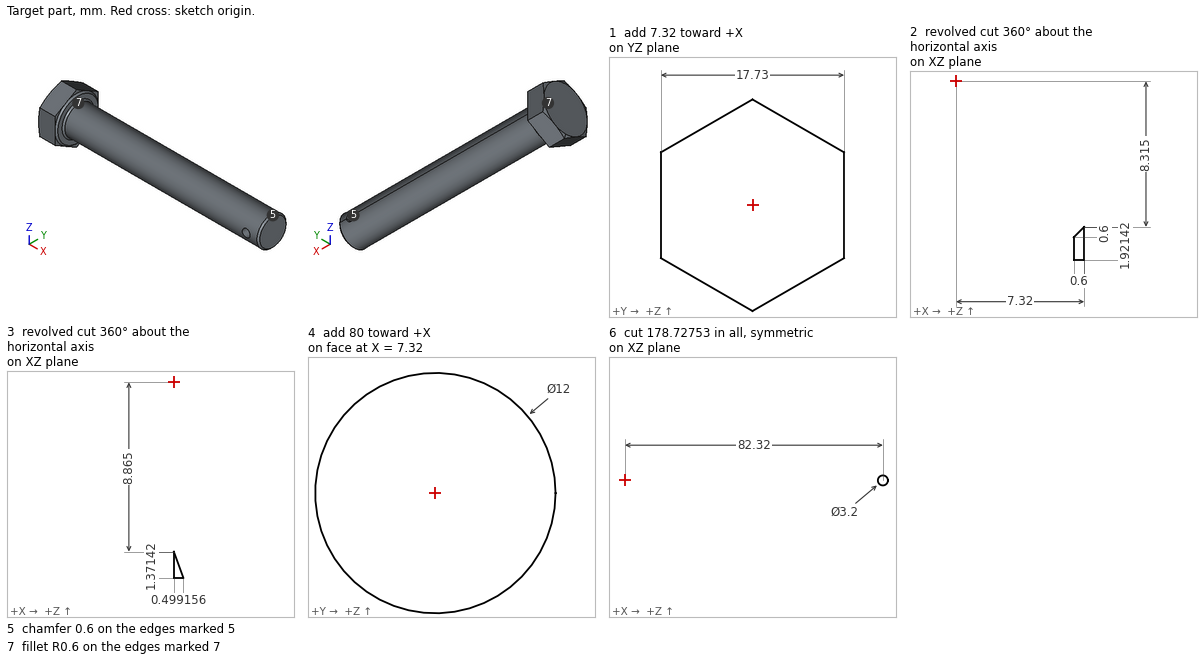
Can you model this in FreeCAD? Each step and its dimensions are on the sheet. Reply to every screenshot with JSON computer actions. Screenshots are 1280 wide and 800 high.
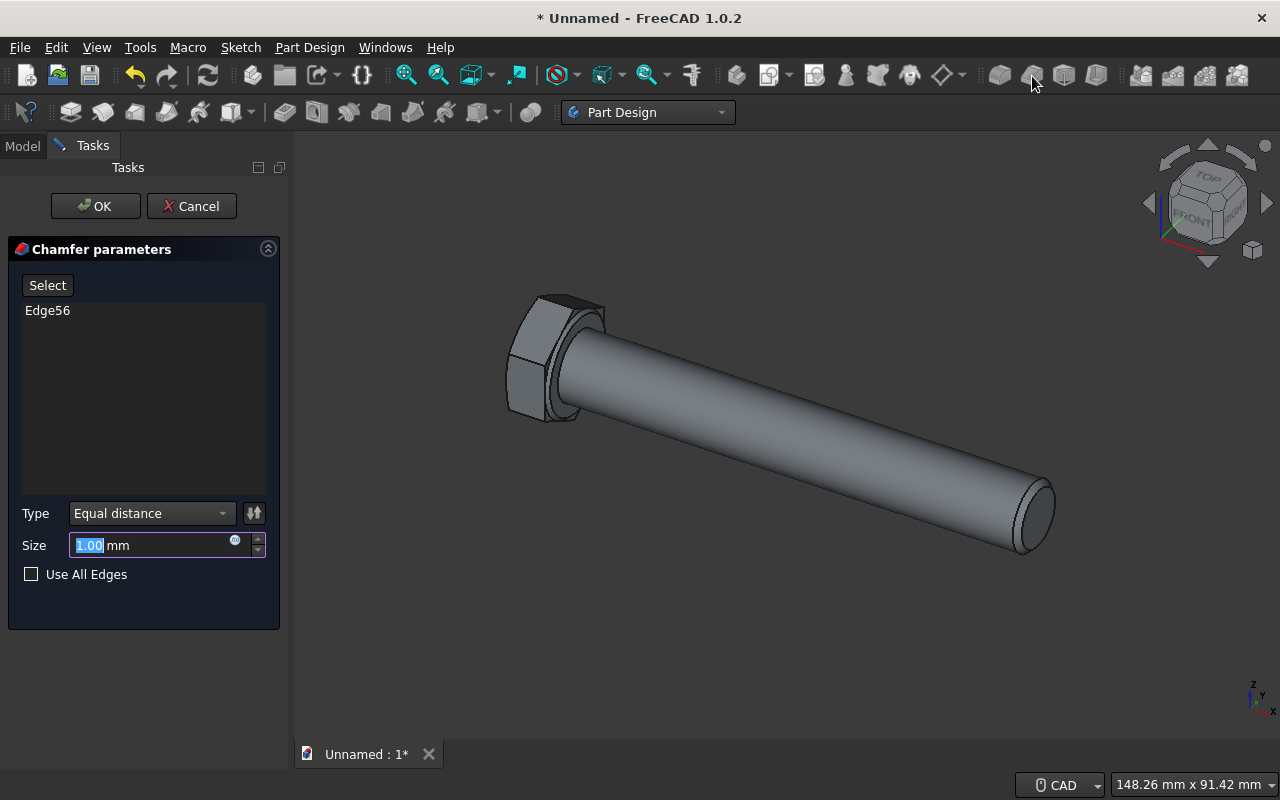
{"action": "type", "text": "0.6"}
{"action": "key", "text": "Tab"}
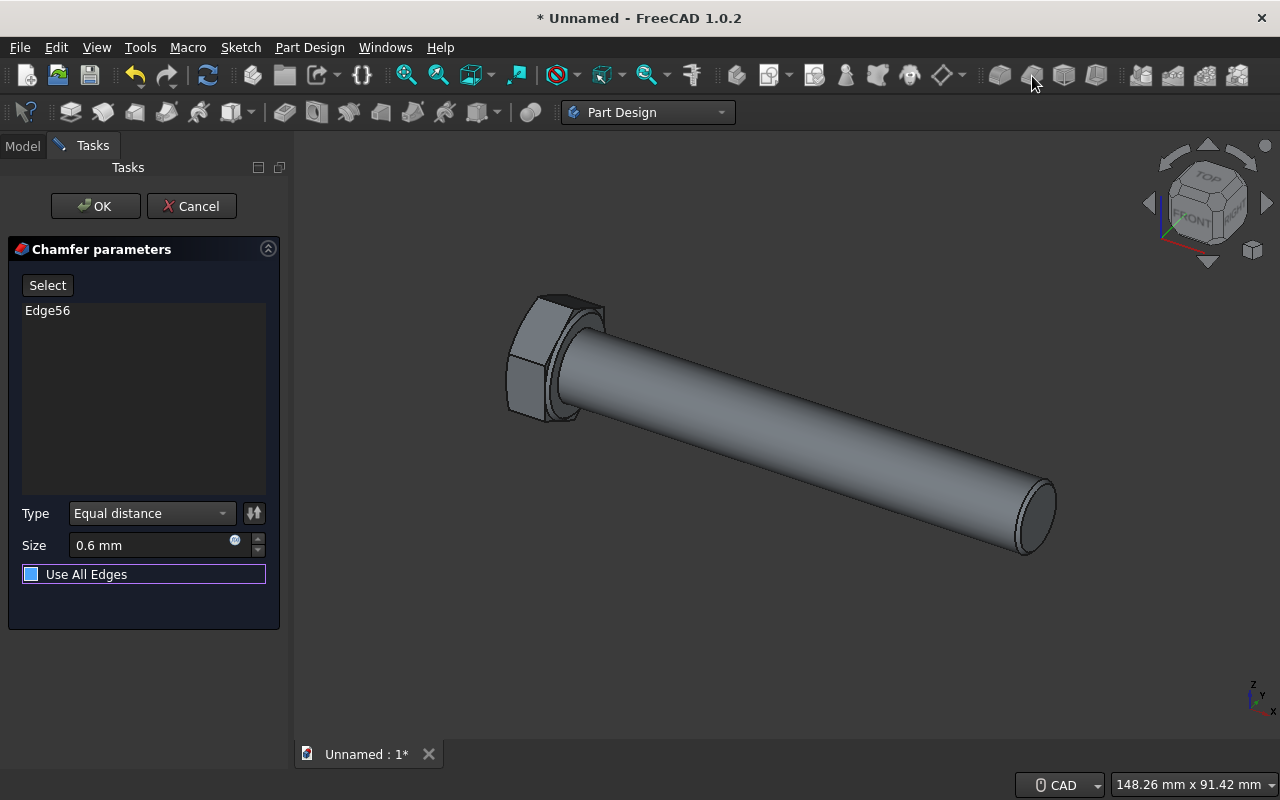
{"action": "left_click", "coordinate": [96, 206]}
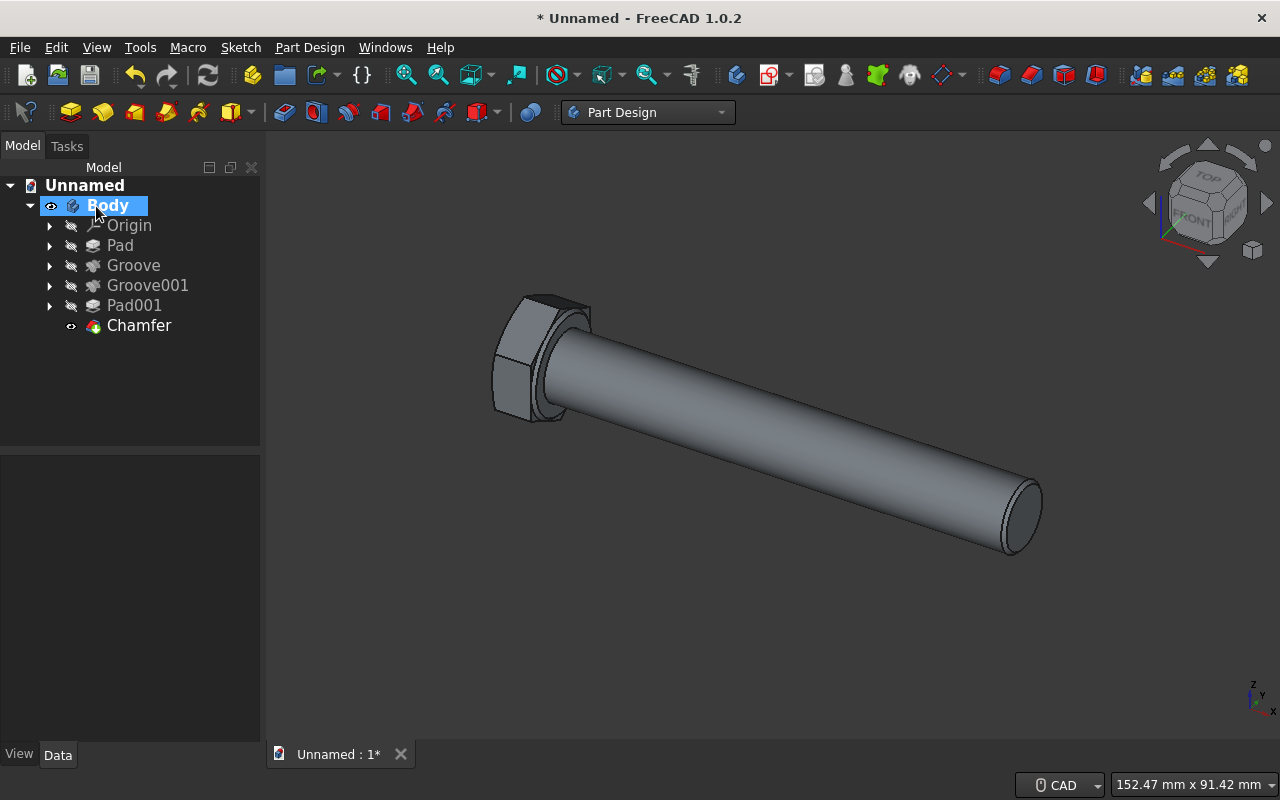
{"action": "left_click", "coordinate": [770, 76]}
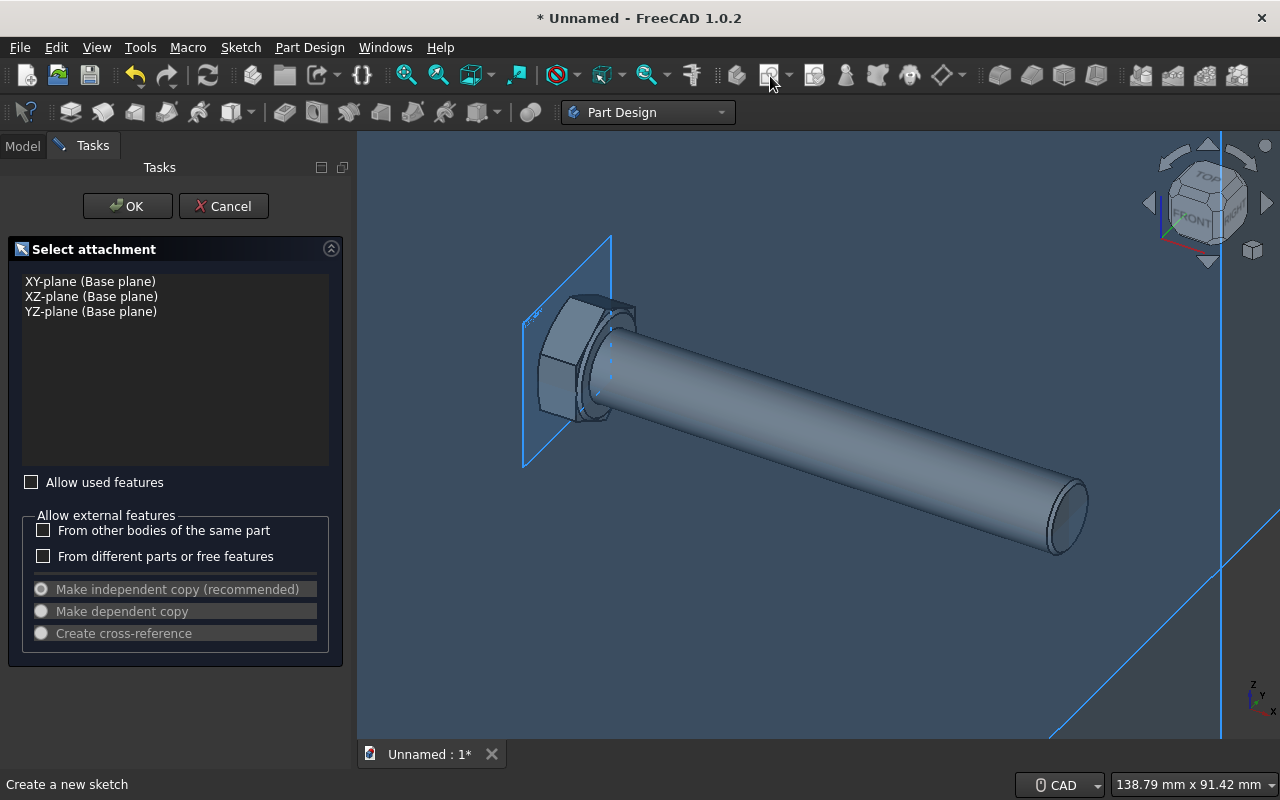
{"action": "left_click", "coordinate": [82, 296]}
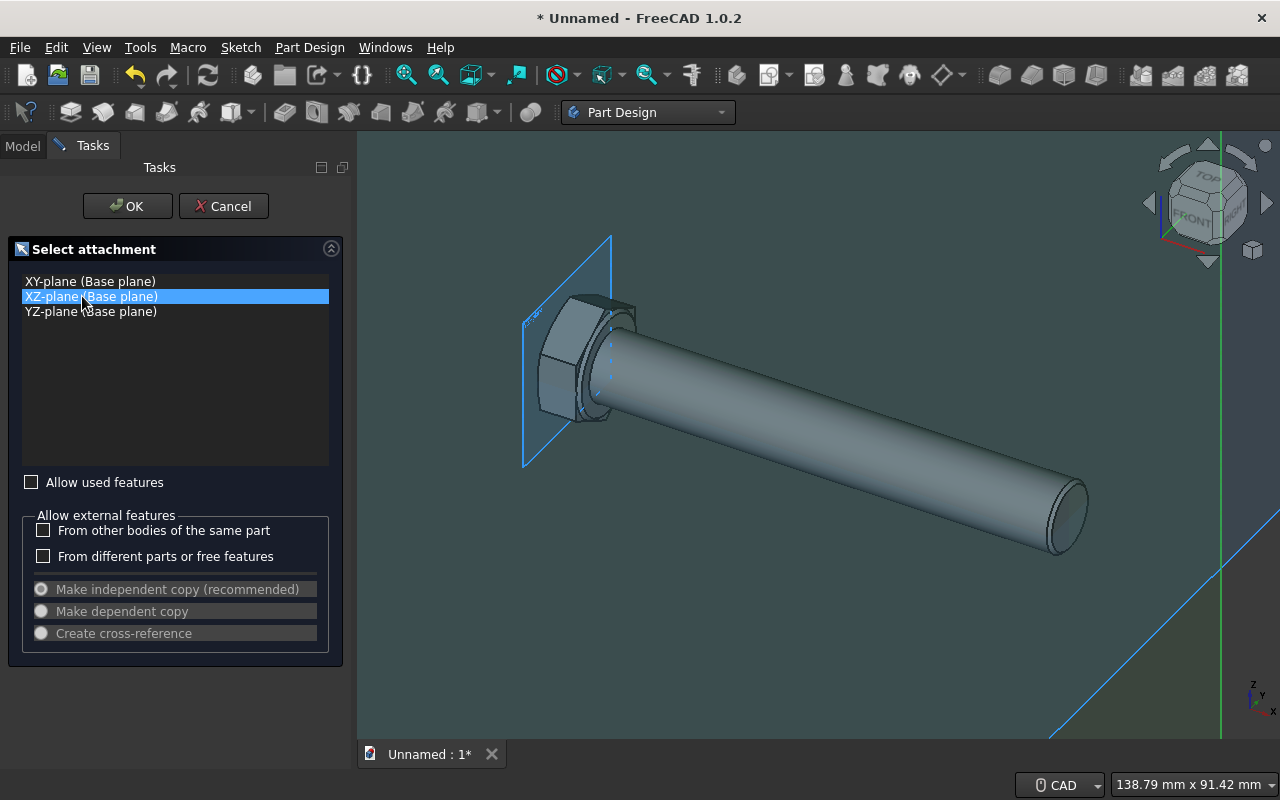
{"action": "left_click", "coordinate": [128, 206]}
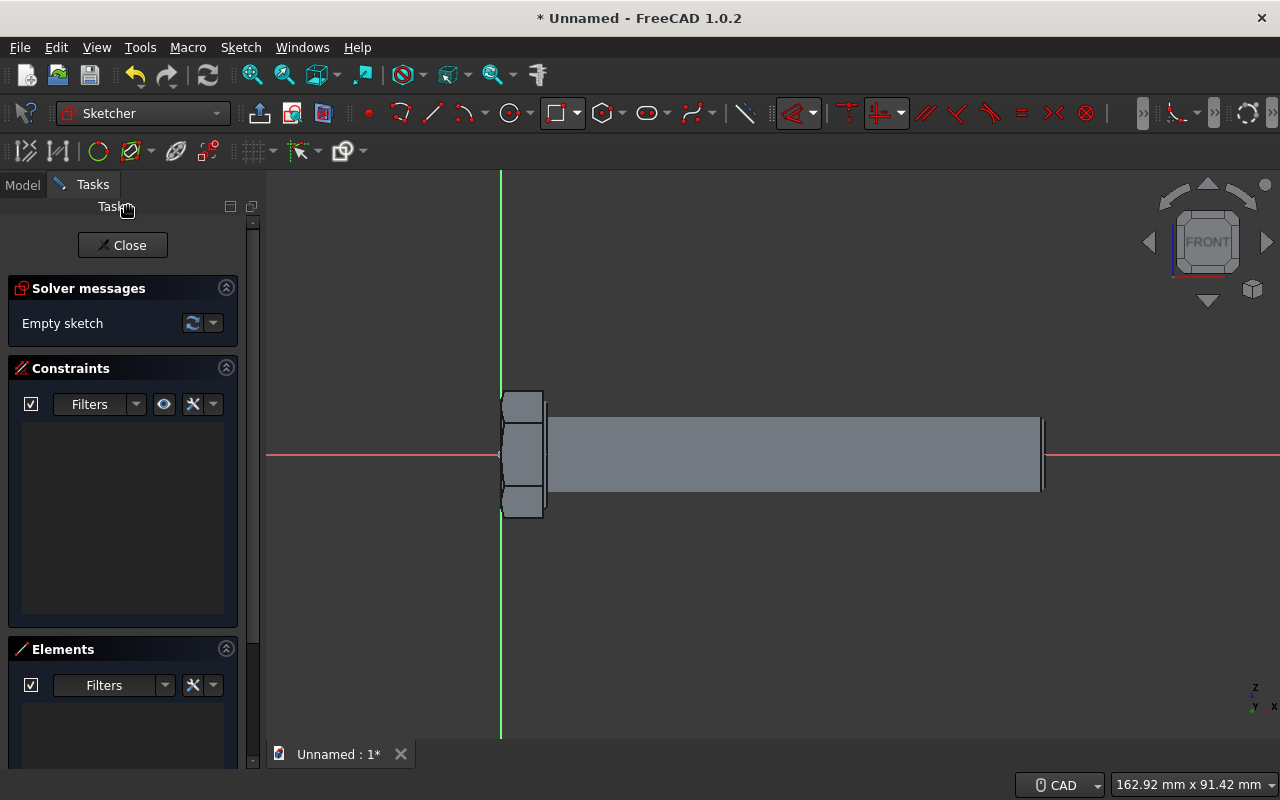
{"action": "left_click", "coordinate": [324, 114]}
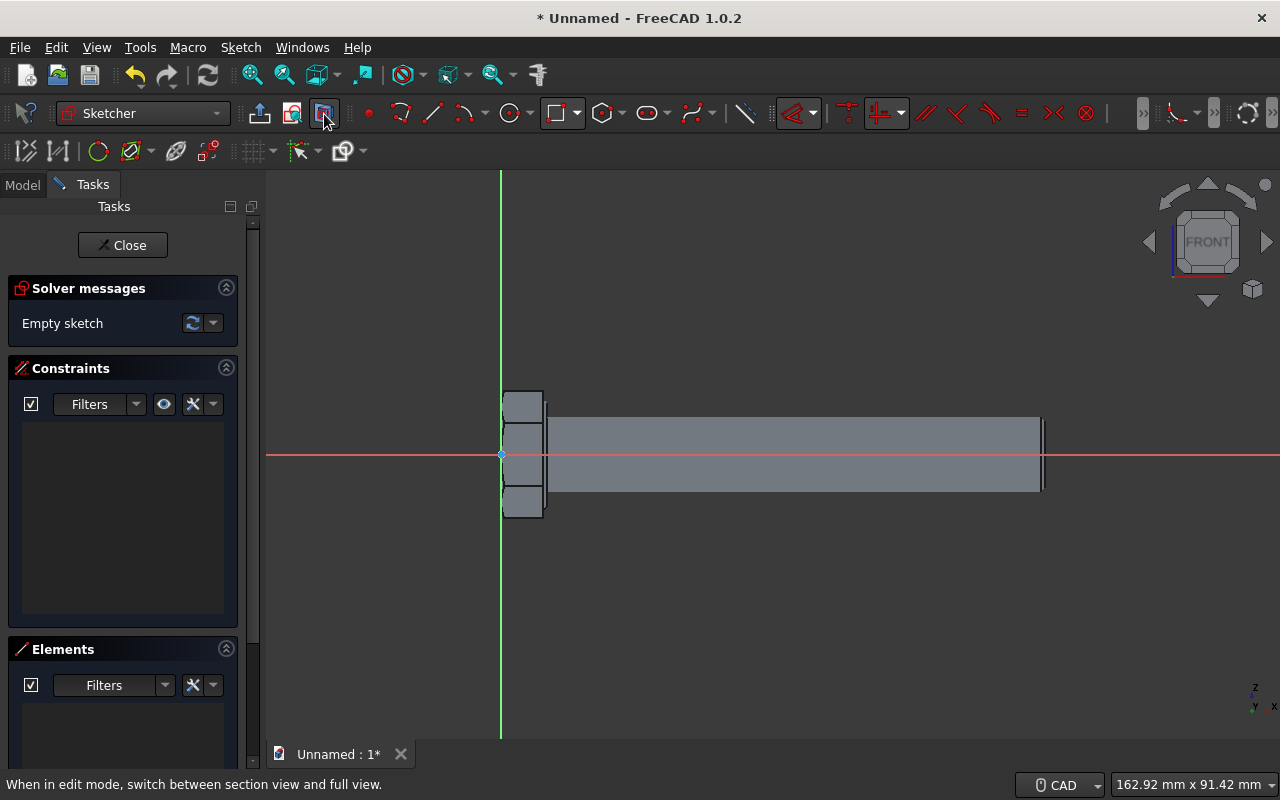
{"action": "scroll", "coordinate": [1030, 455], "scroll_direction": "up", "scroll_amount": 15}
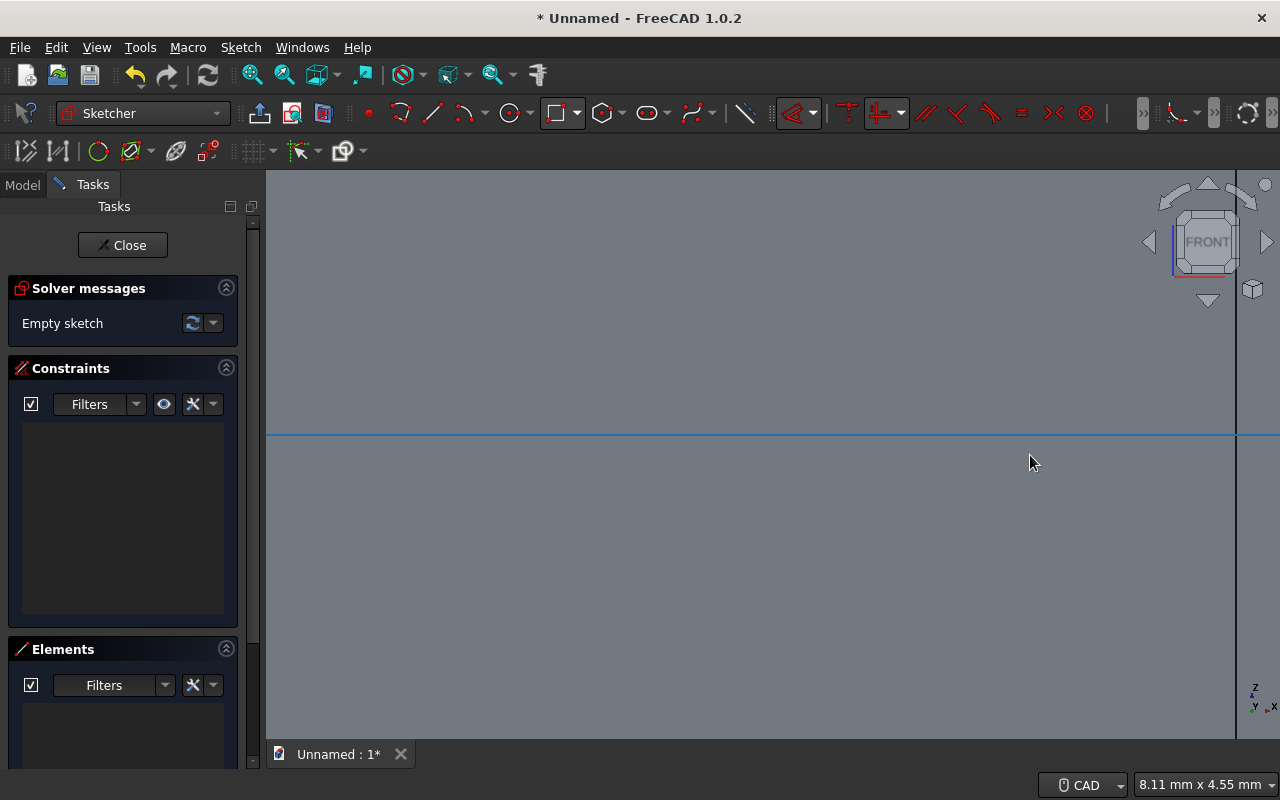
{"action": "left_click", "coordinate": [510, 114]}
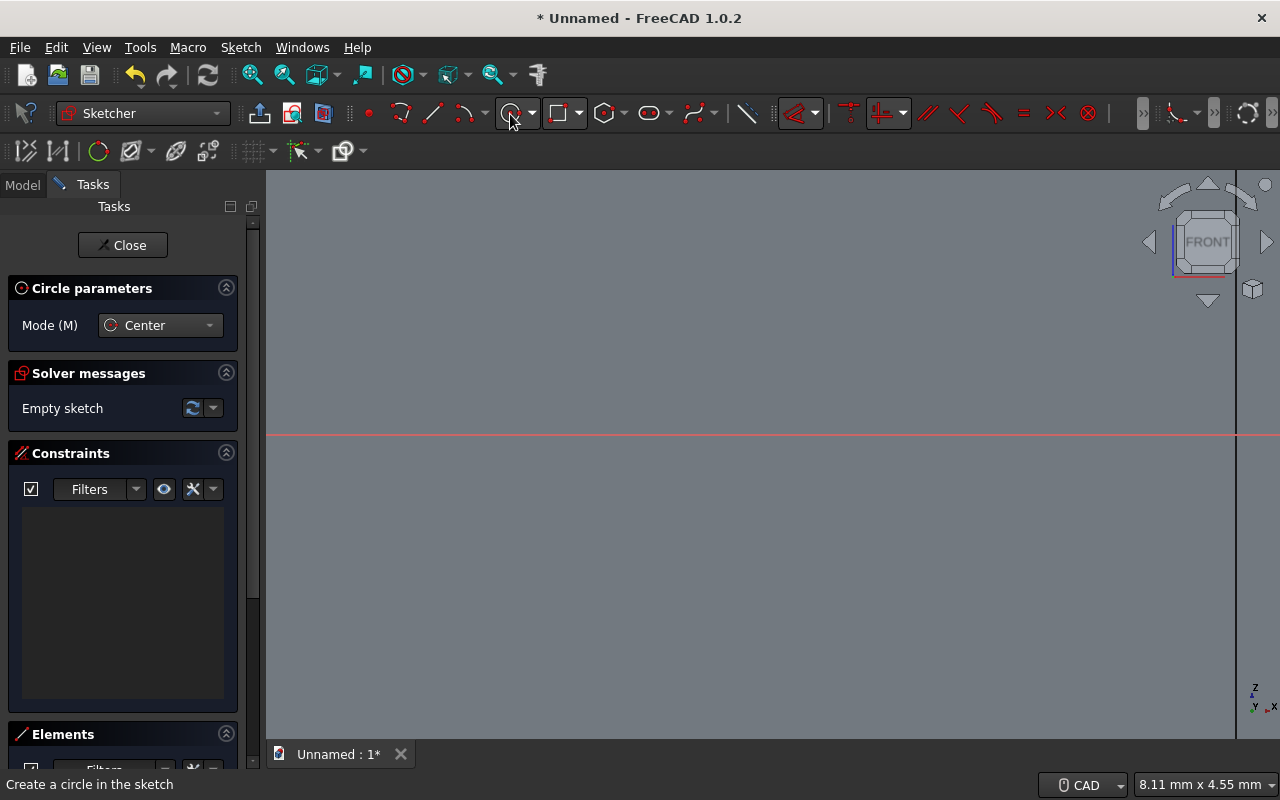
{"action": "left_click", "coordinate": [686, 435]}
{"action": "left_click", "coordinate": [828, 294]}
{"action": "key", "text": "Escape"}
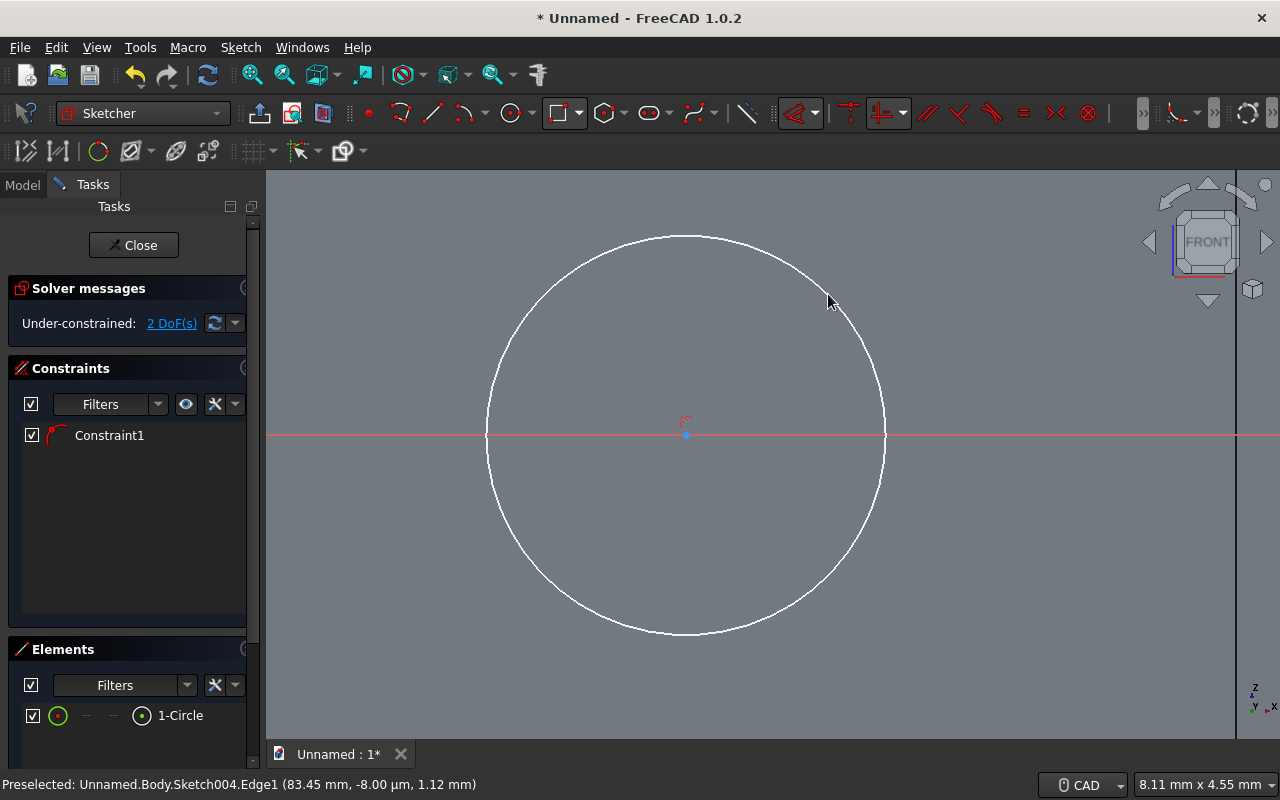
{"action": "left_click", "coordinate": [827, 294]}